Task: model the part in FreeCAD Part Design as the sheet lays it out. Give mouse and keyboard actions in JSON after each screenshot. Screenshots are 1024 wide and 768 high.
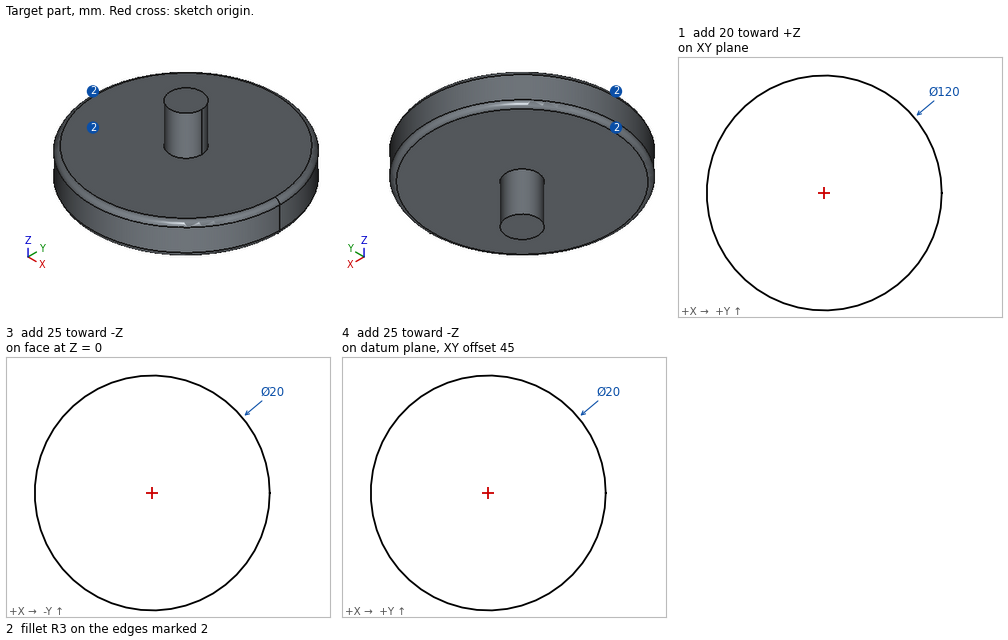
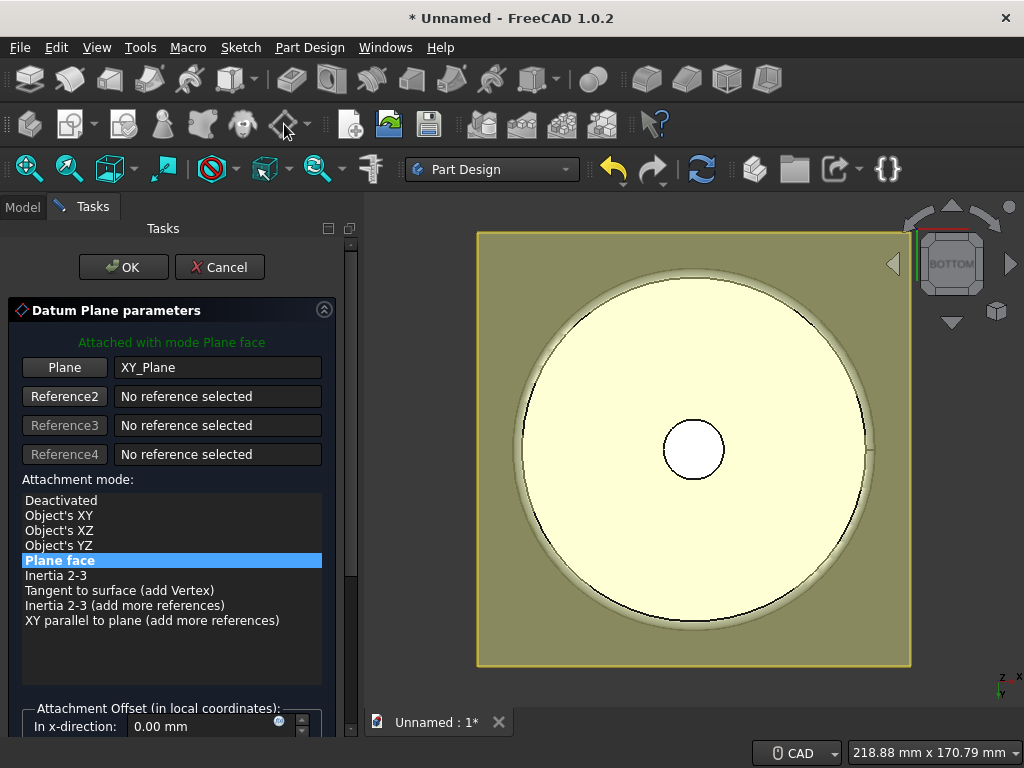
{"action": "scroll", "coordinate": [351, 487], "scroll_direction": "down", "scroll_amount": 3}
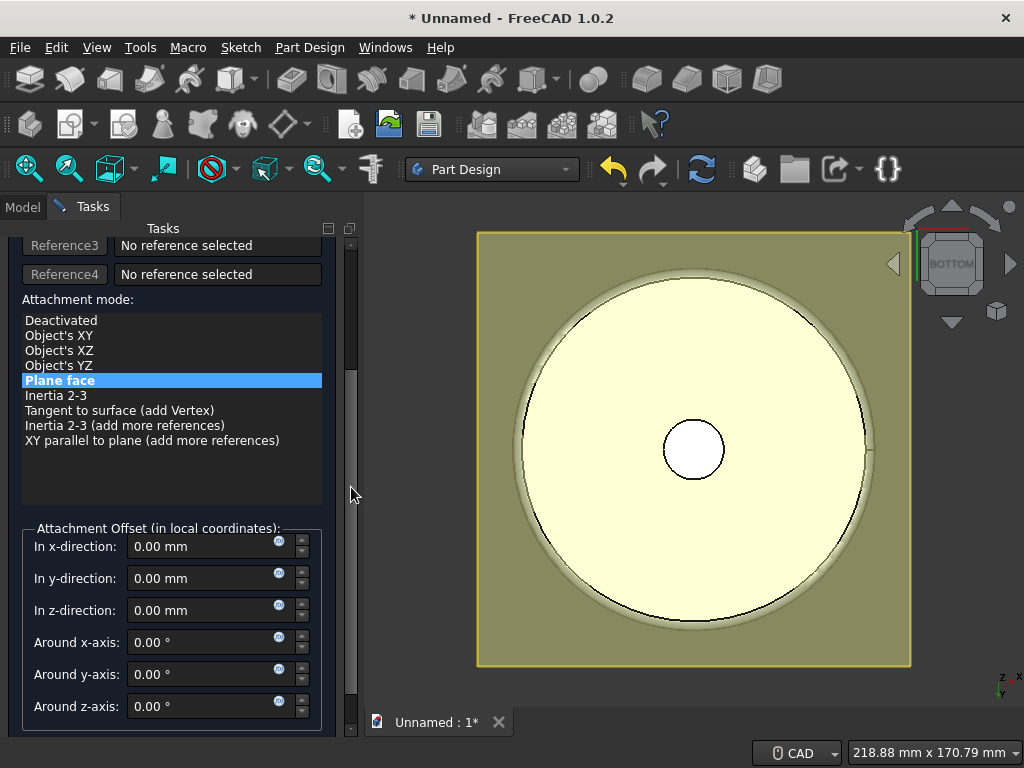
{"action": "triple_click", "coordinate": [210, 610]}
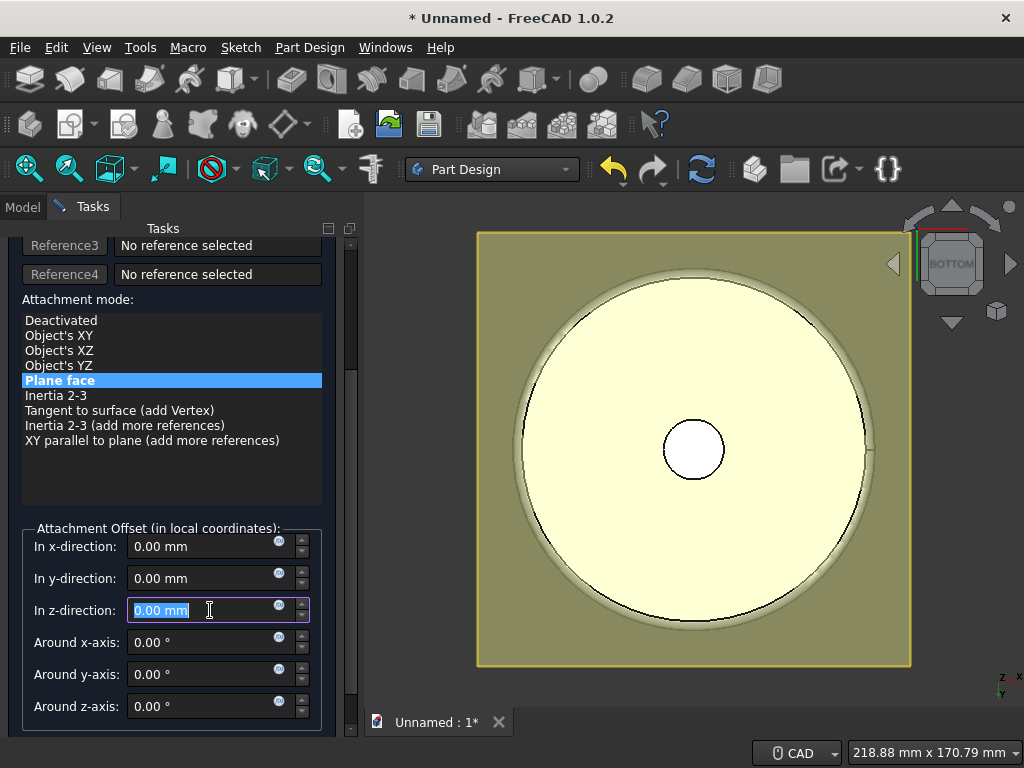
{"action": "type", "text": "45"}
{"action": "key", "text": "Tab"}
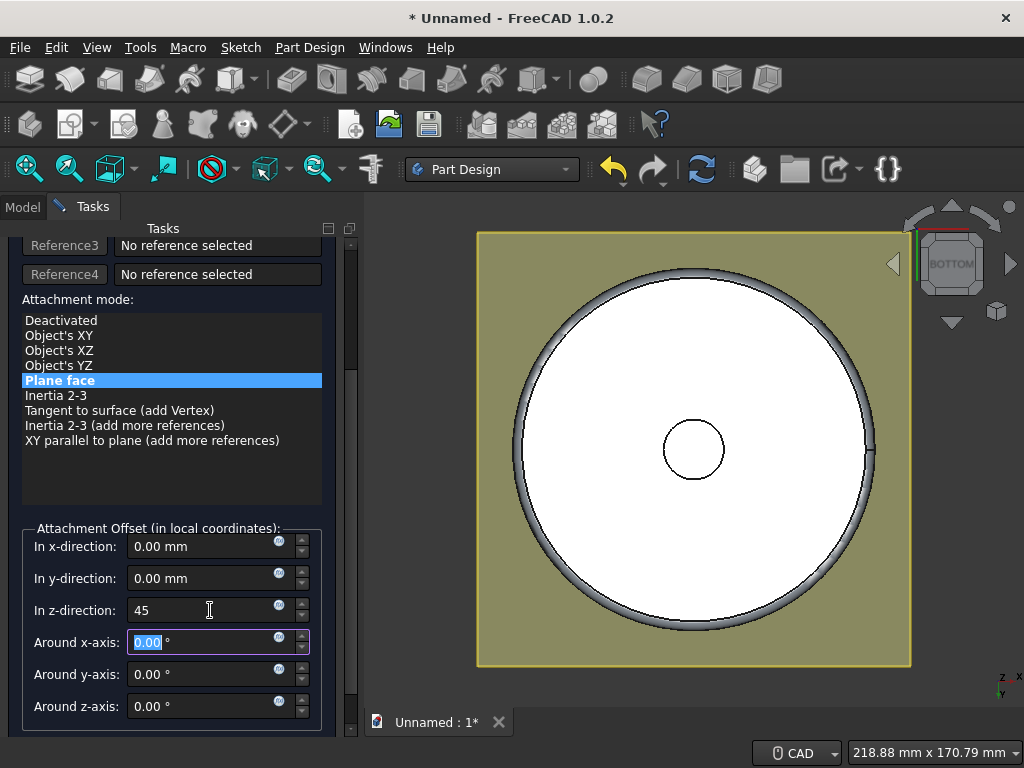
{"action": "scroll", "coordinate": [351, 487], "scroll_direction": "up", "scroll_amount": 4}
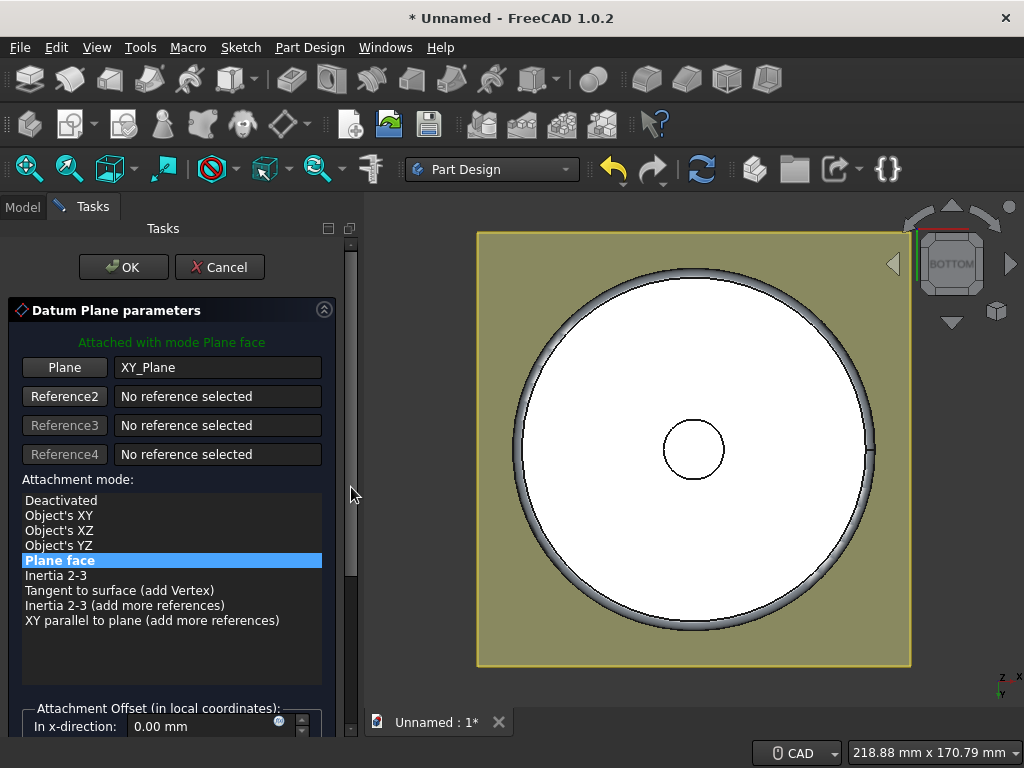
{"action": "left_click", "coordinate": [124, 267]}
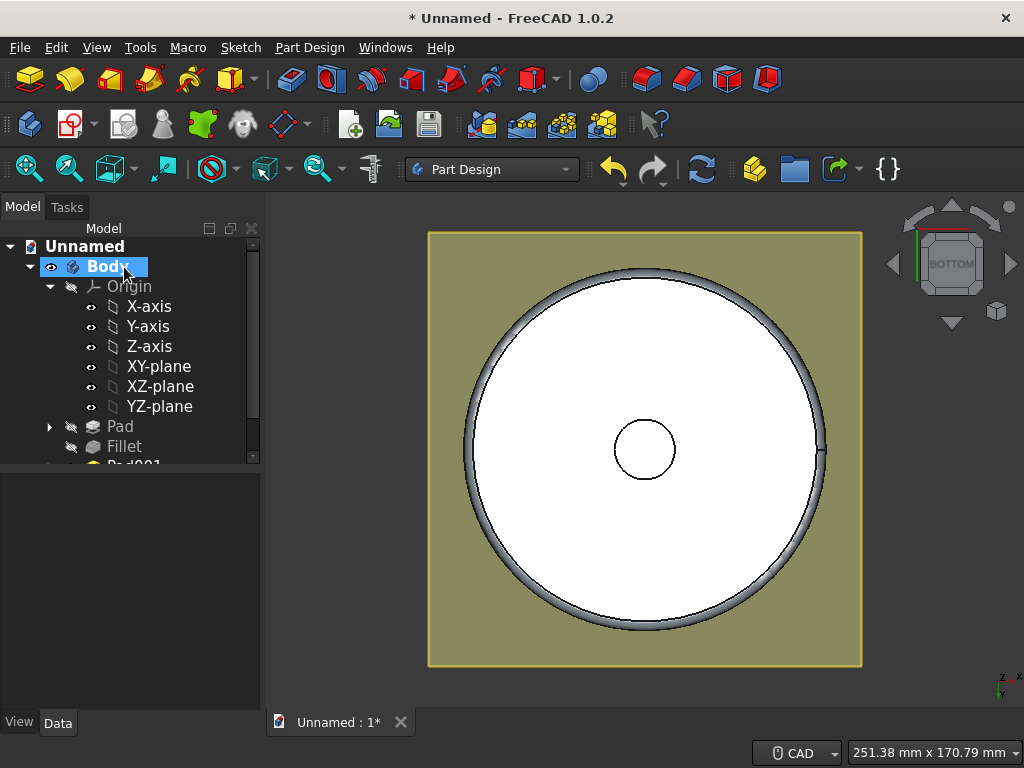
{"action": "scroll", "coordinate": [100, 342], "scroll_direction": "down", "scroll_amount": 3}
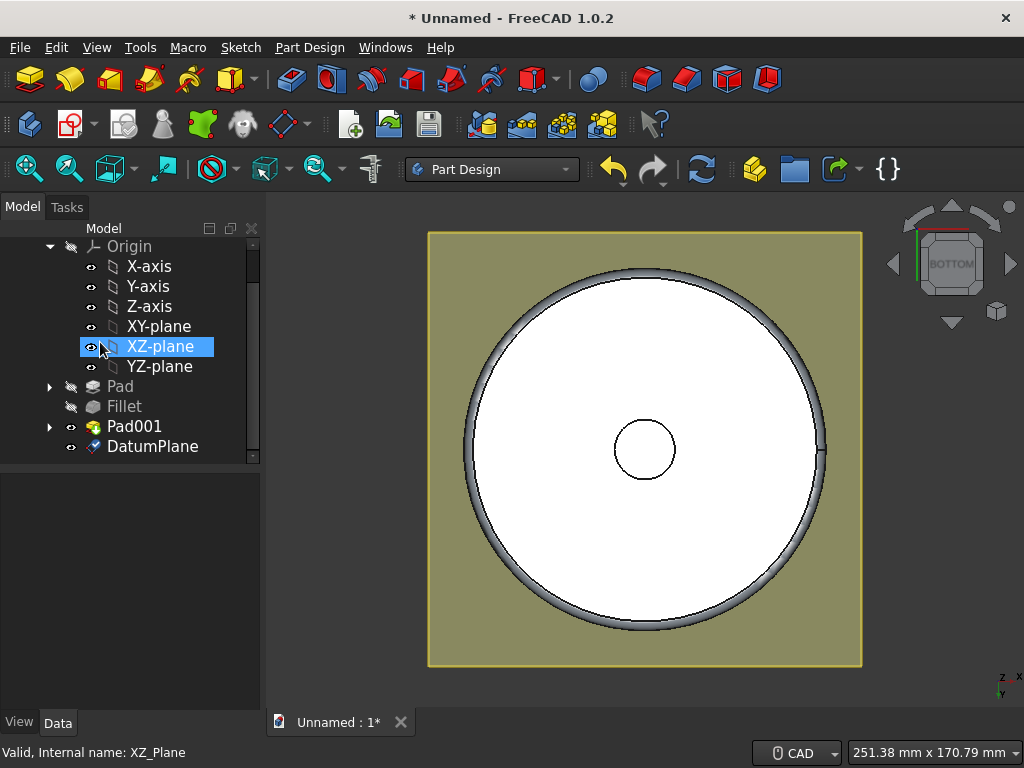
{"action": "left_click", "coordinate": [116, 447]}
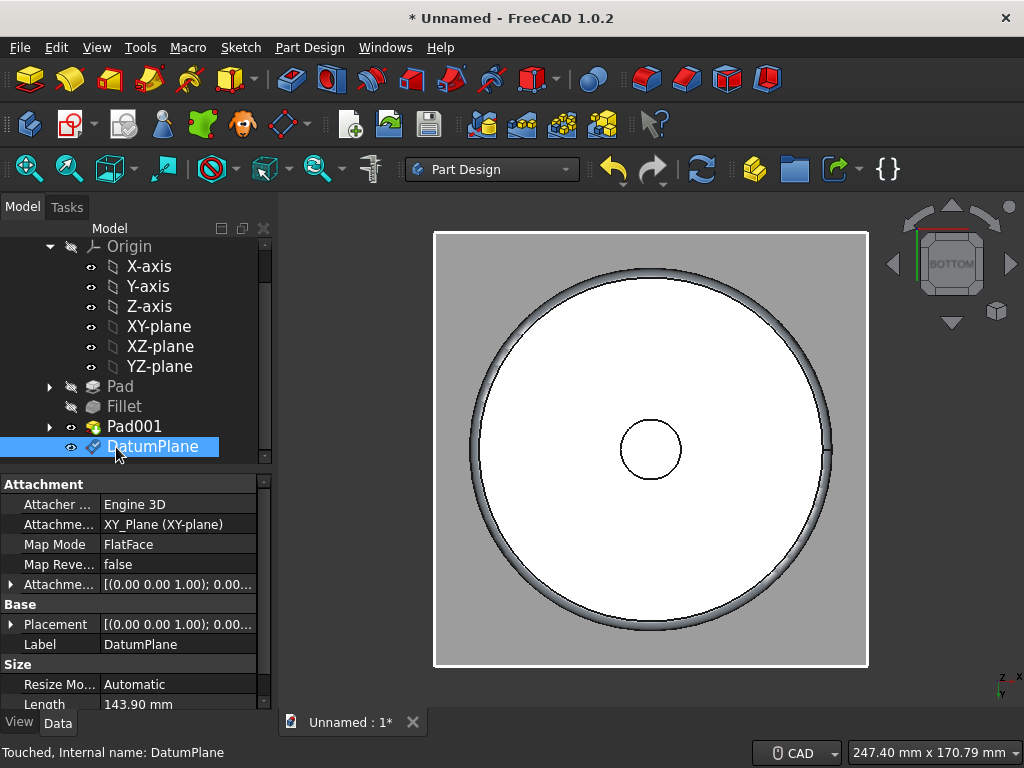
{"action": "left_click", "coordinate": [70, 124]}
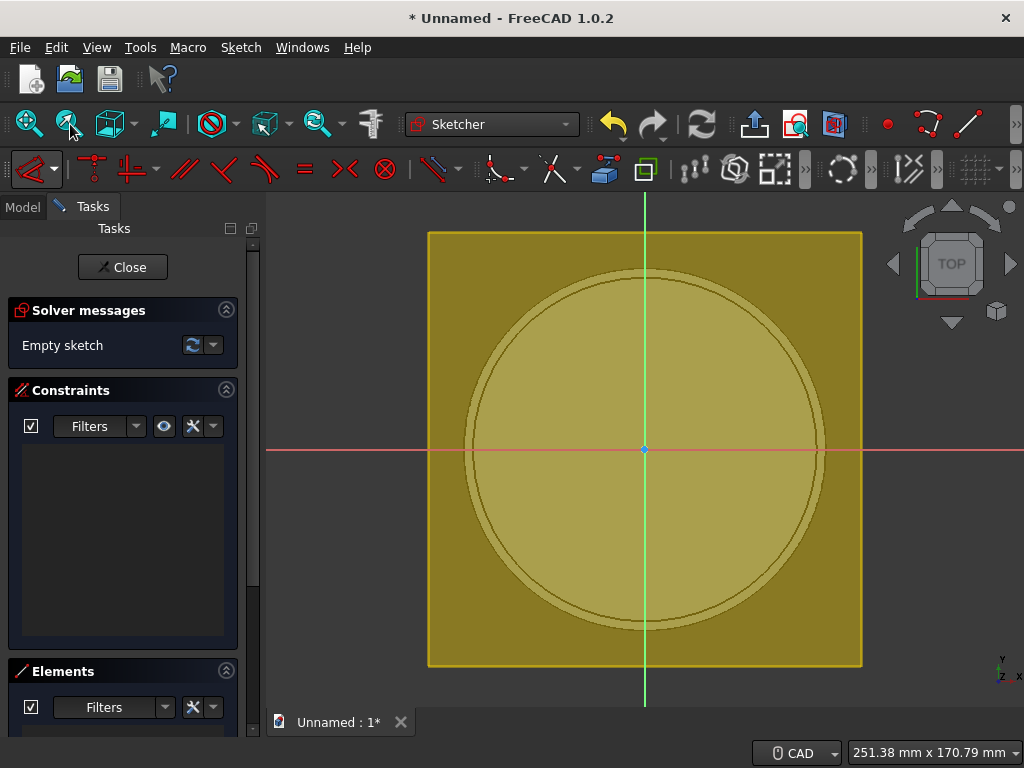
{"action": "scroll", "coordinate": [662, 449], "scroll_direction": "up", "scroll_amount": 8}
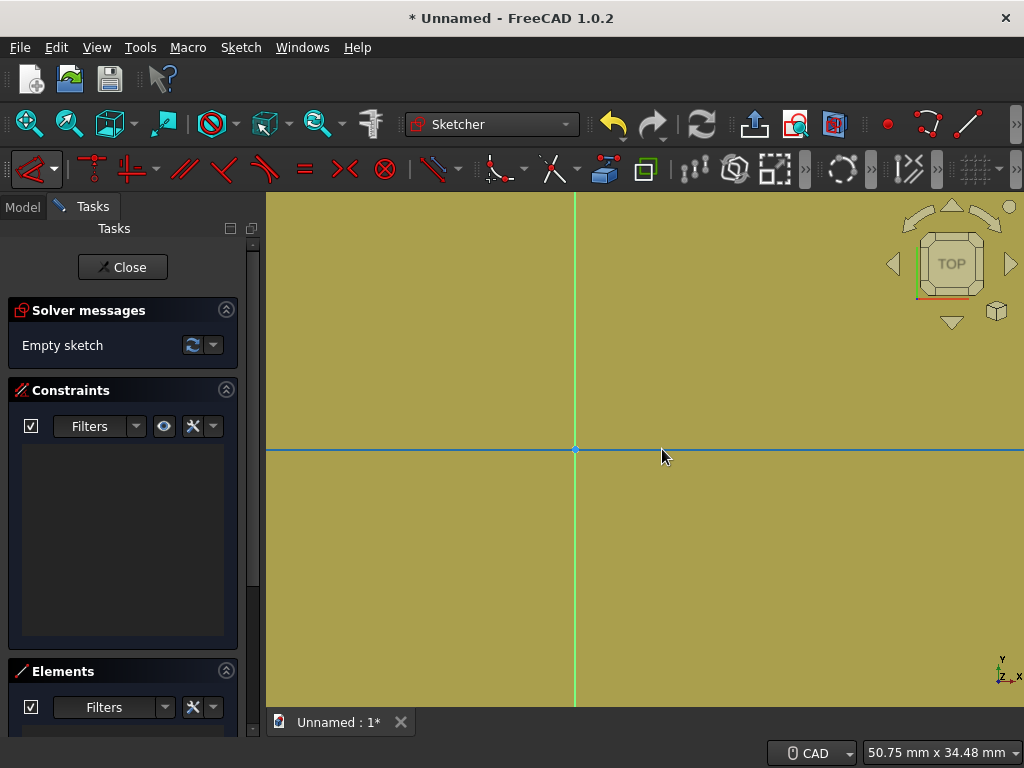
{"action": "key", "text": "g c"}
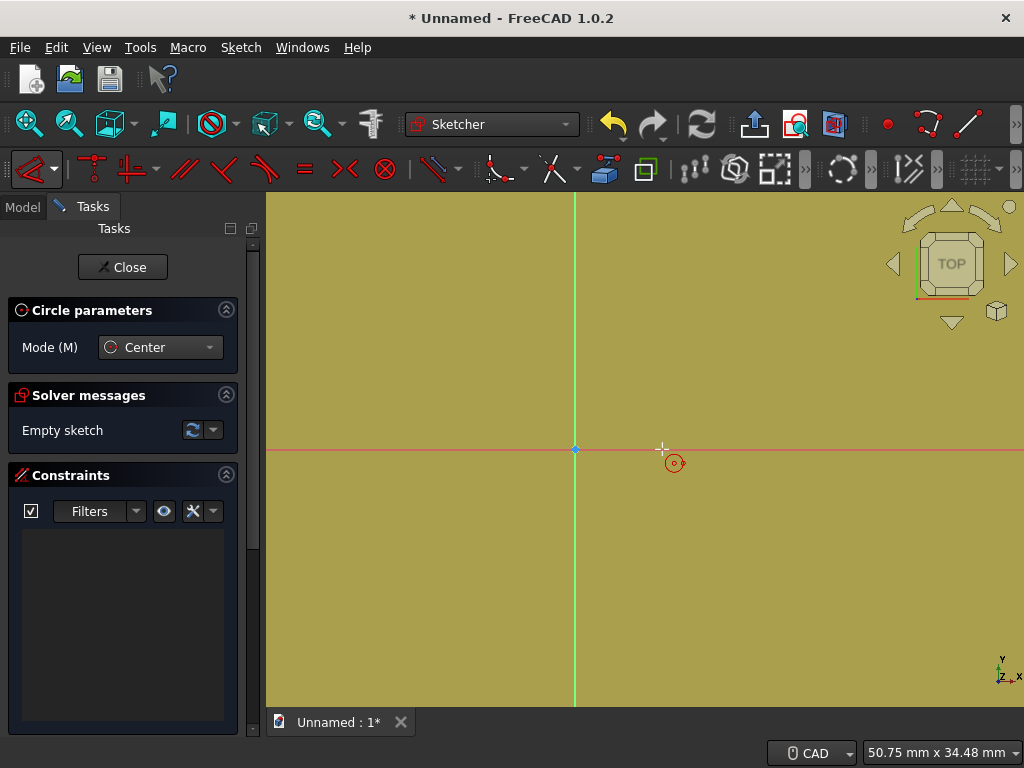
{"action": "left_click", "coordinate": [575, 449]}
{"action": "left_click", "coordinate": [681, 344]}
{"action": "key", "text": "Escape"}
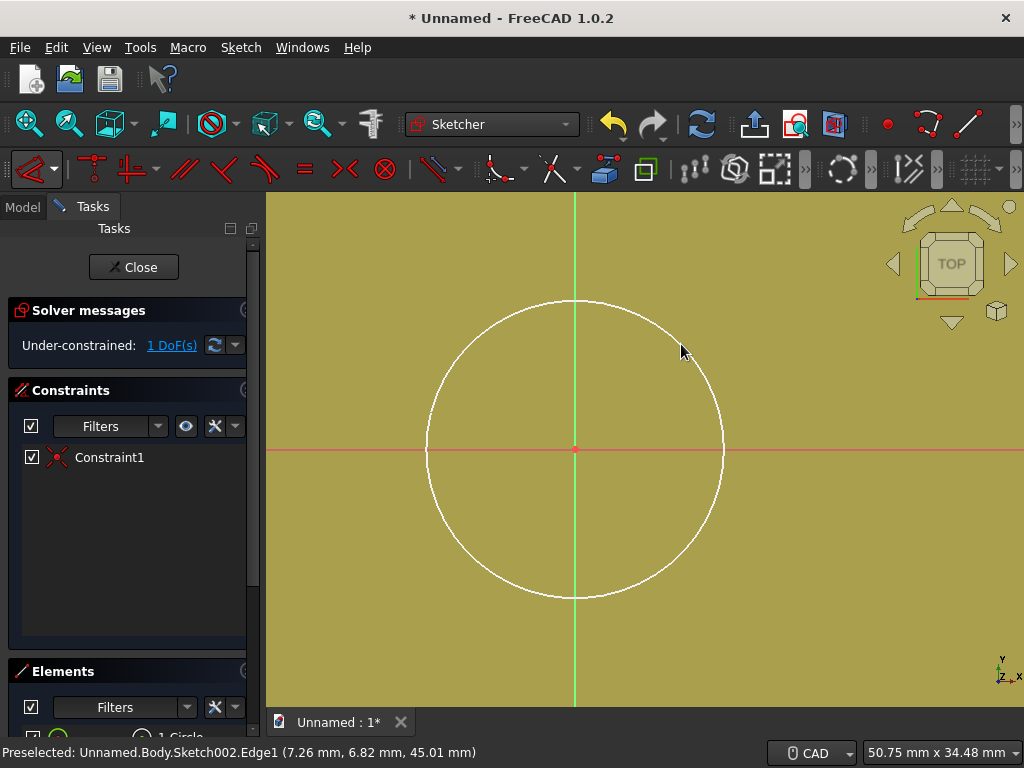
{"action": "left_click", "coordinate": [680, 344]}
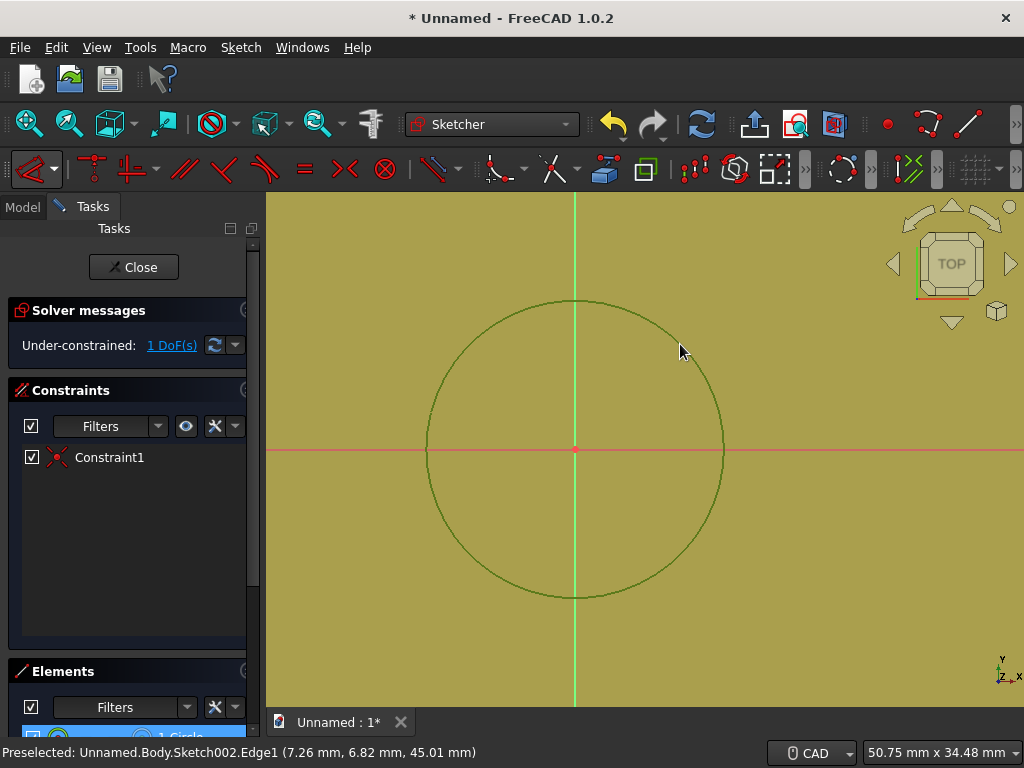
{"action": "key", "text": "k o"}